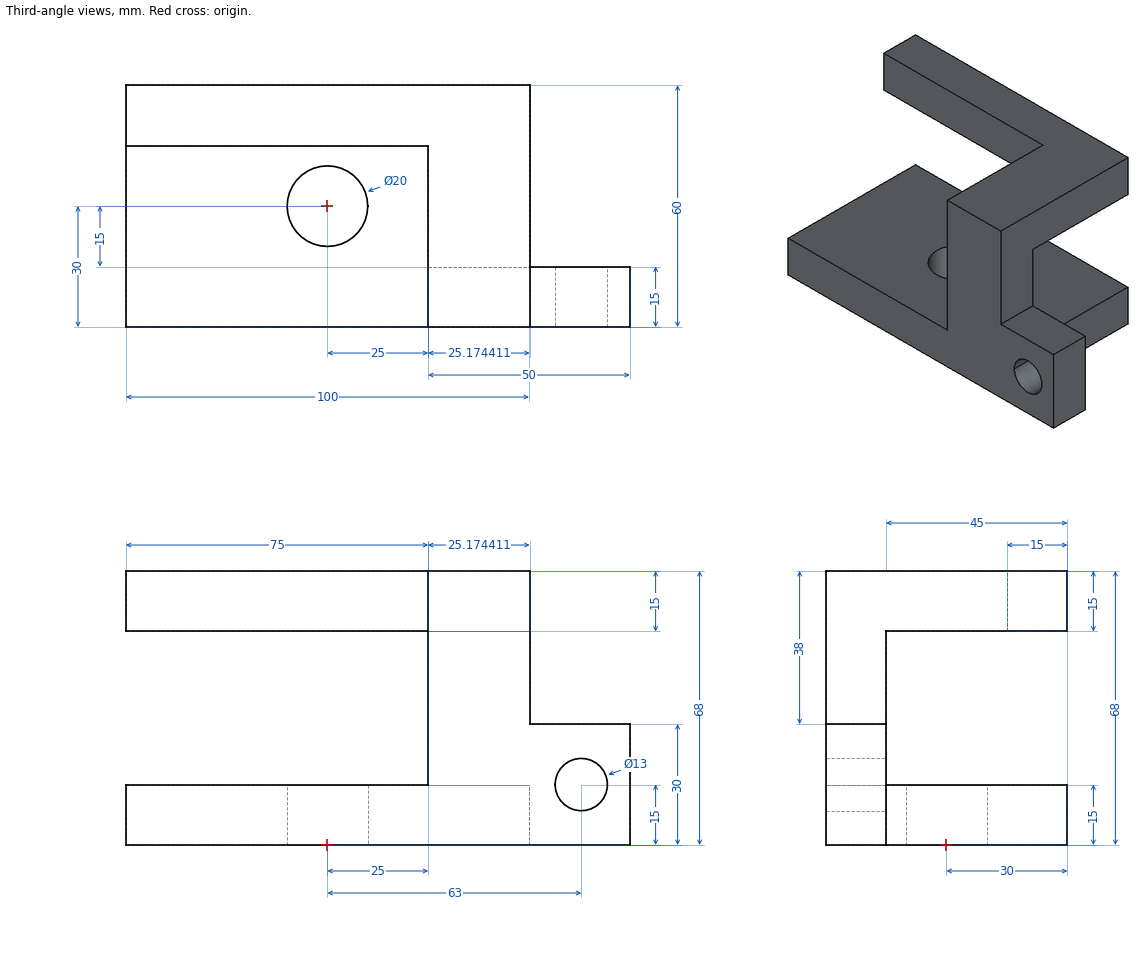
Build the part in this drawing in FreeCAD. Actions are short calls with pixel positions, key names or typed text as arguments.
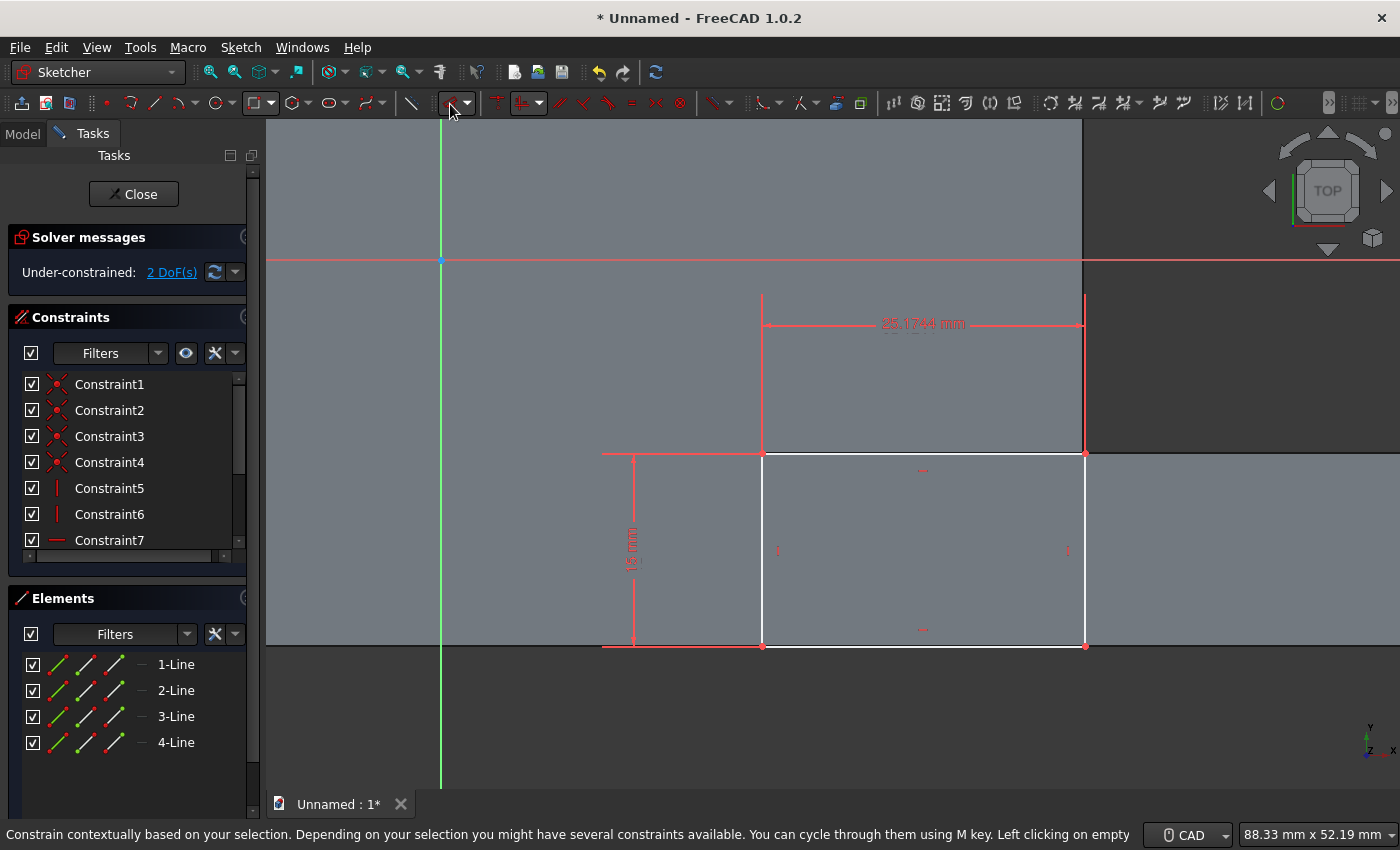
click(762, 454)
click(602, 226)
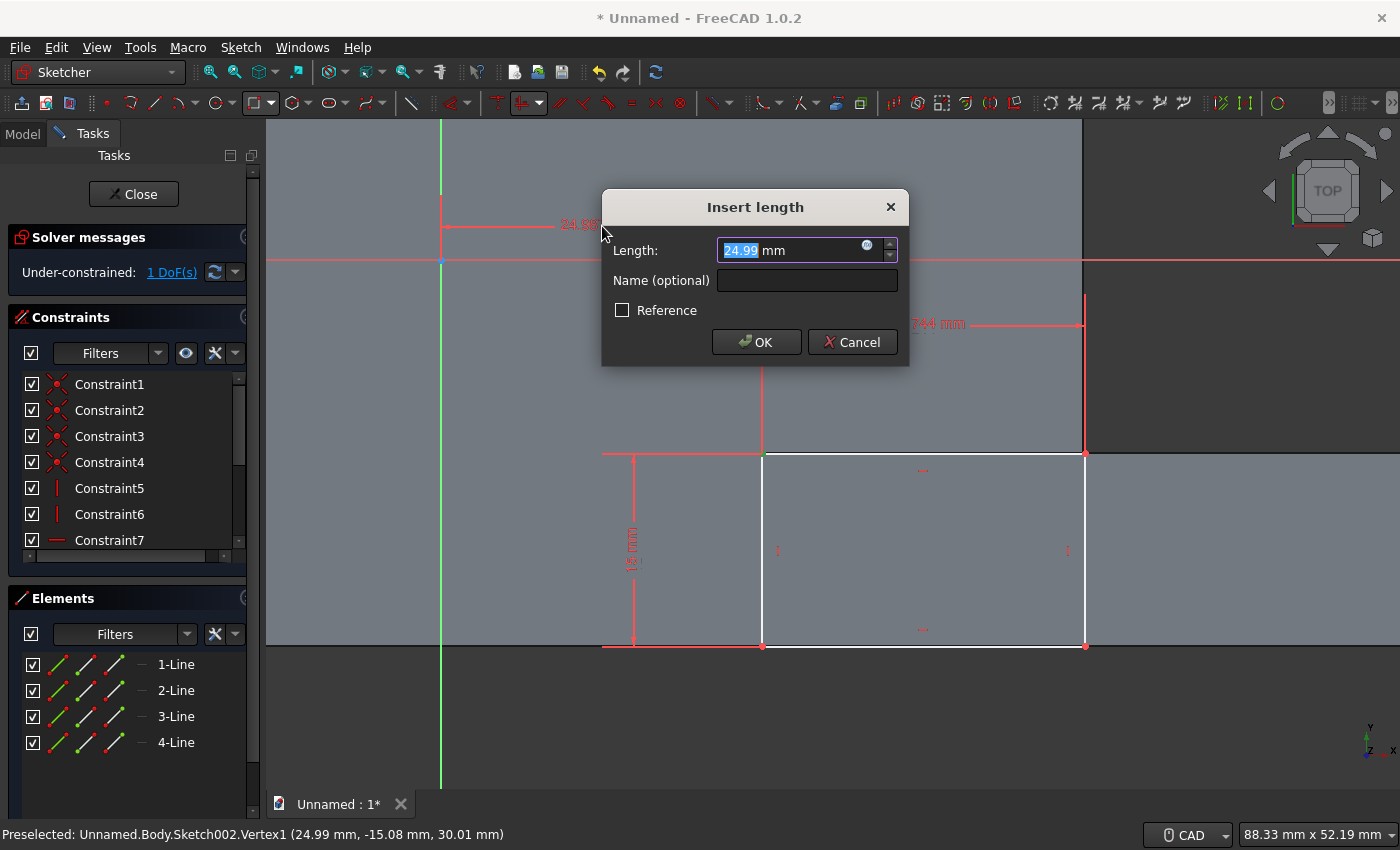
text(25)
key(Return)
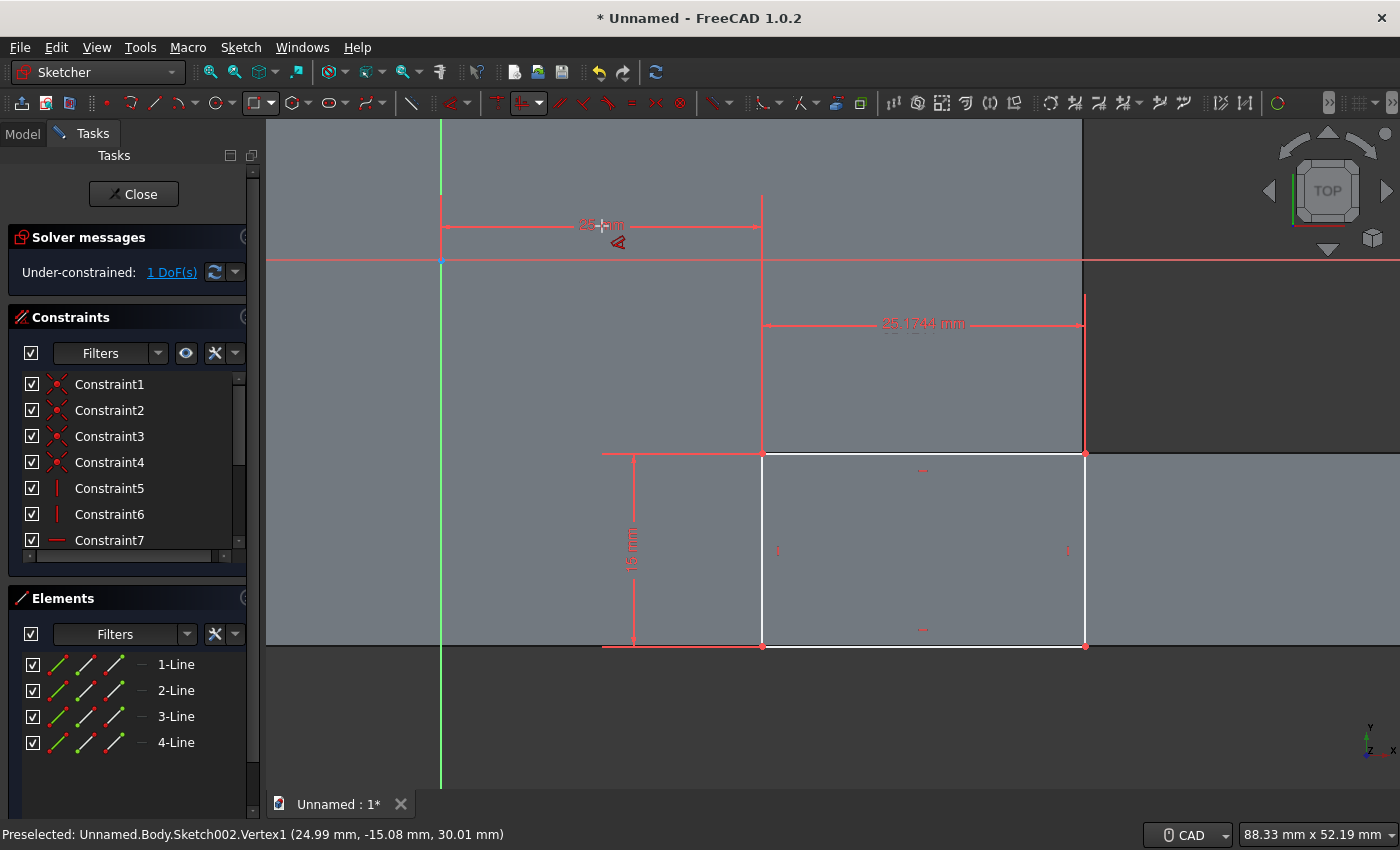
click(762, 454)
click(407, 357)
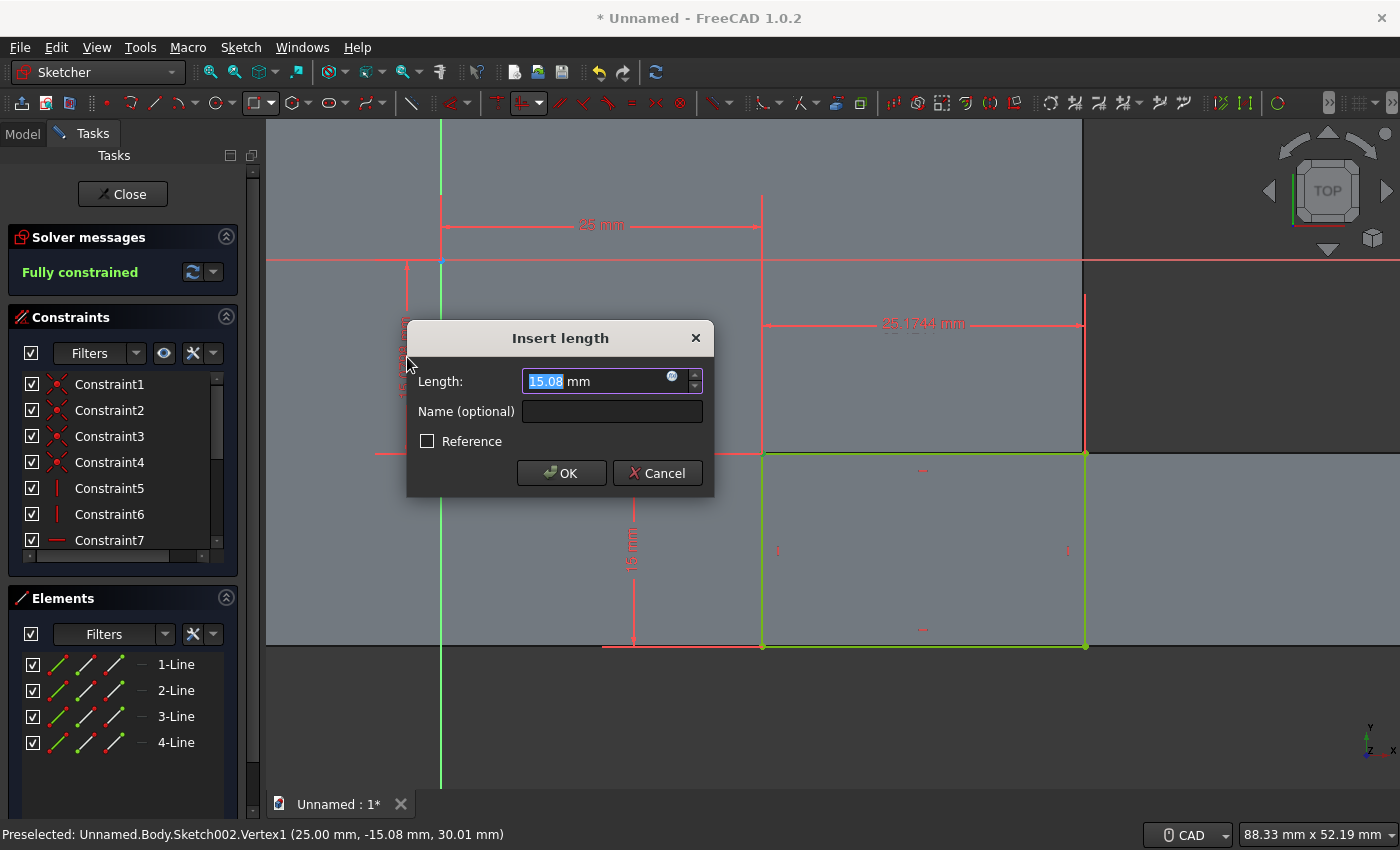
text(15)
key(Return)
key(Escape)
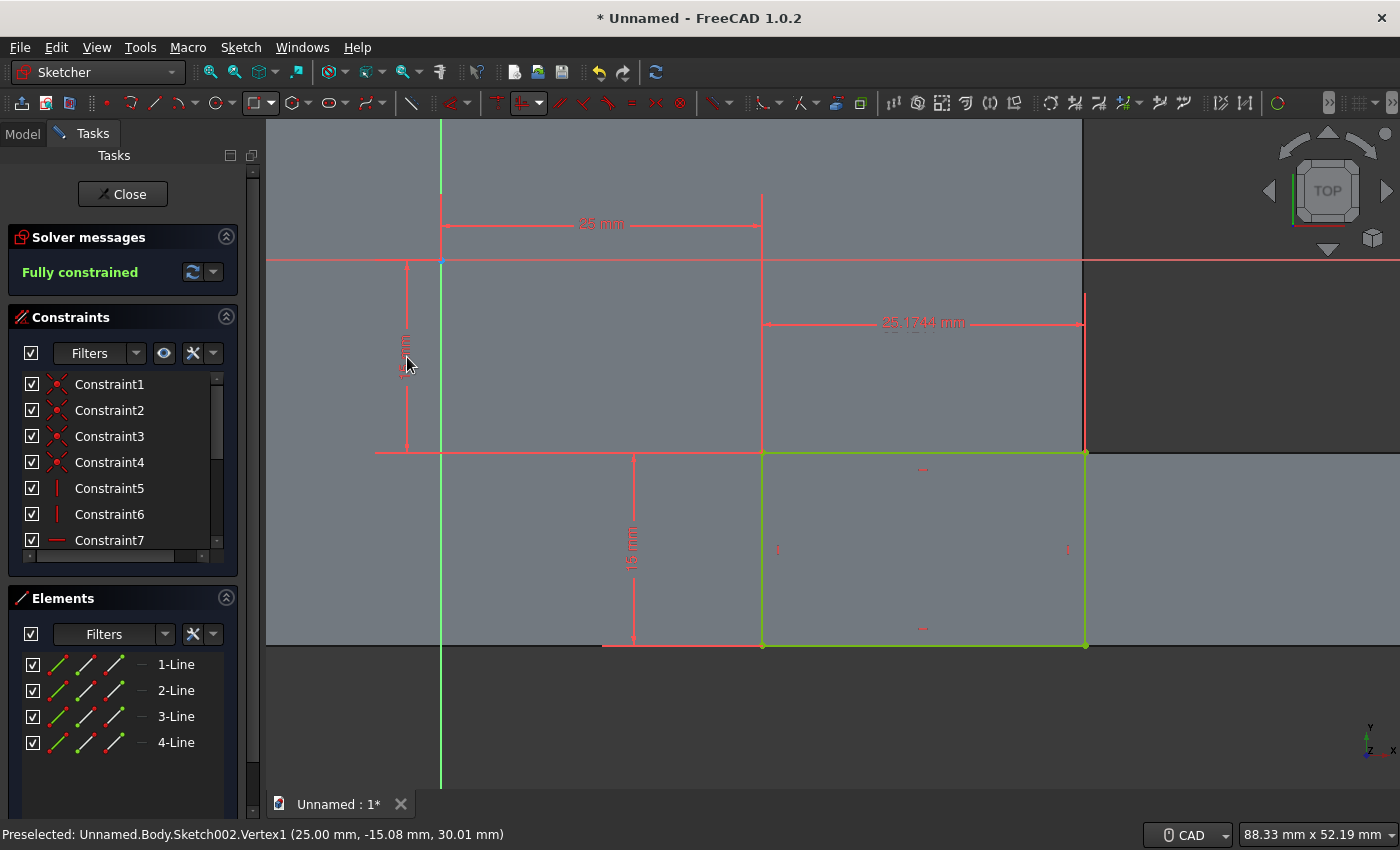
click(123, 194)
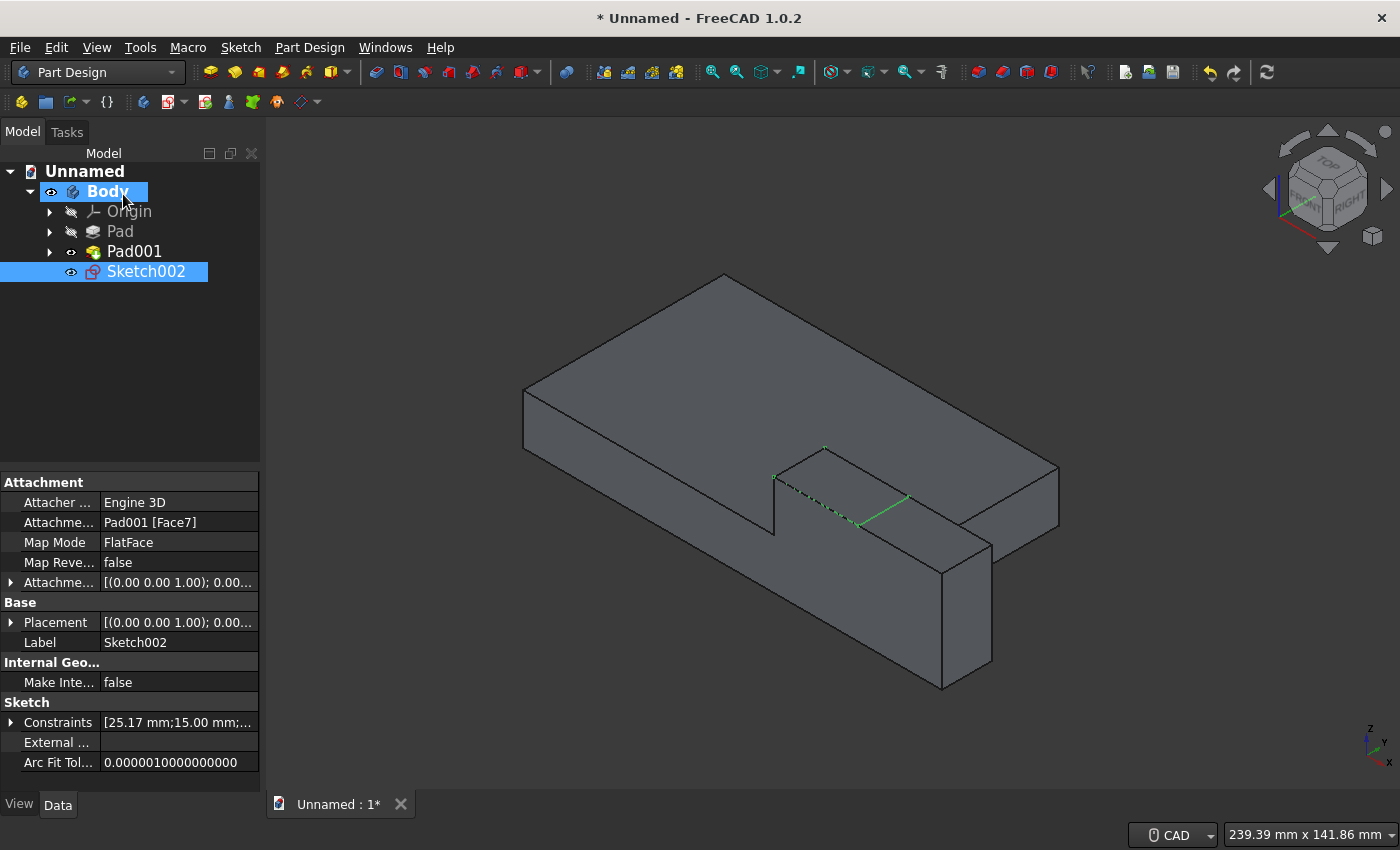
click(212, 72)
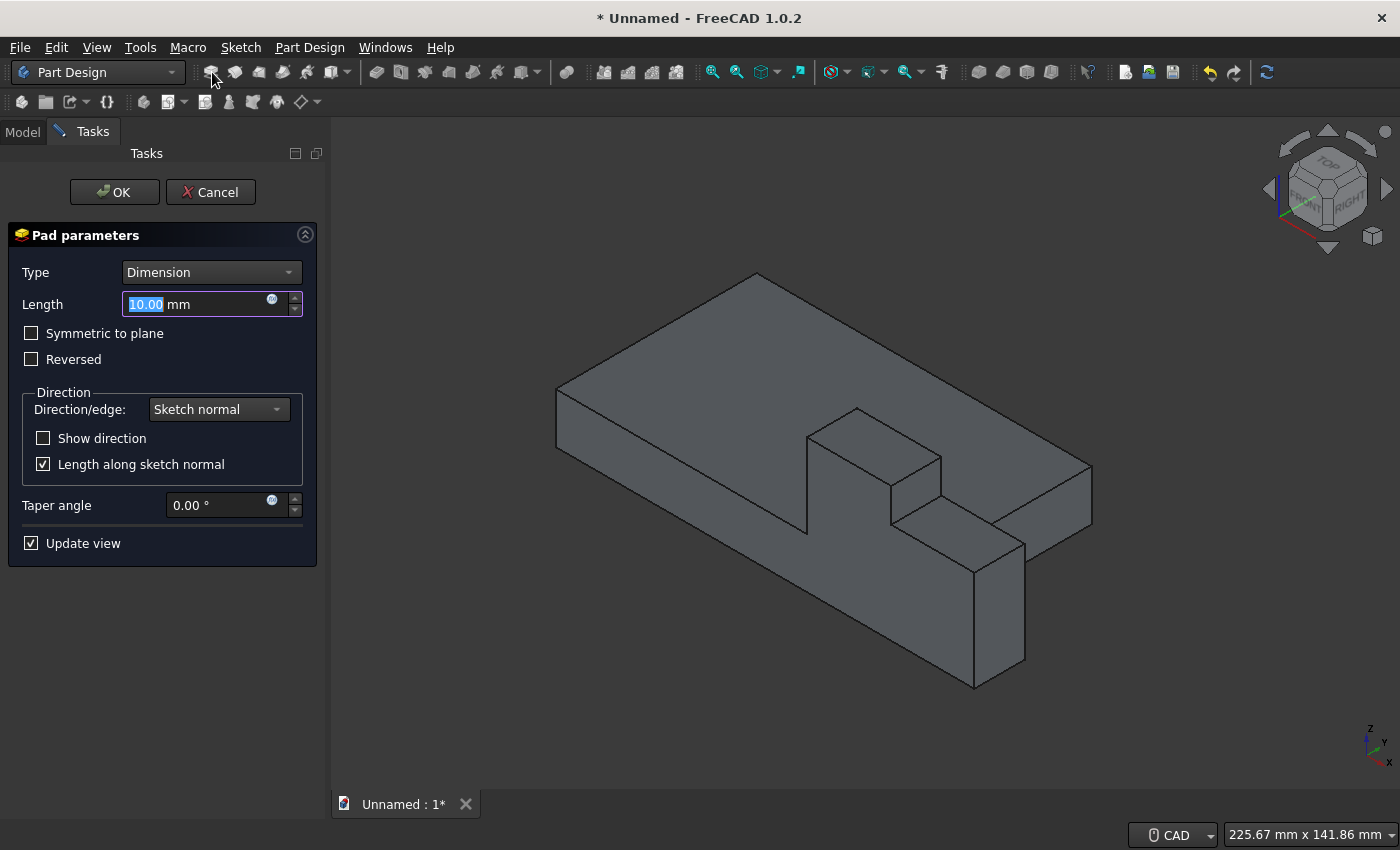
text(38)
key(Tab)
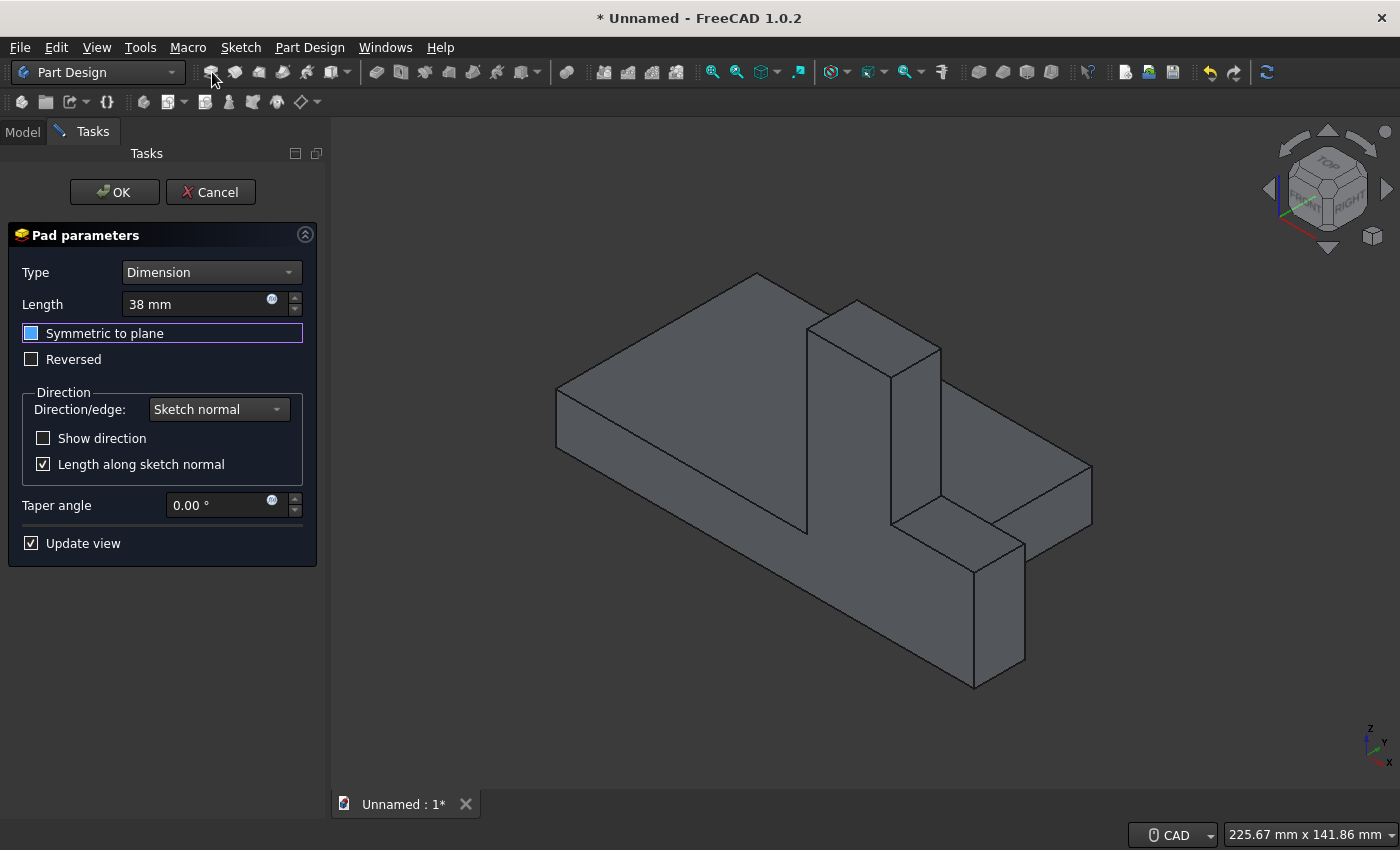
click(115, 192)